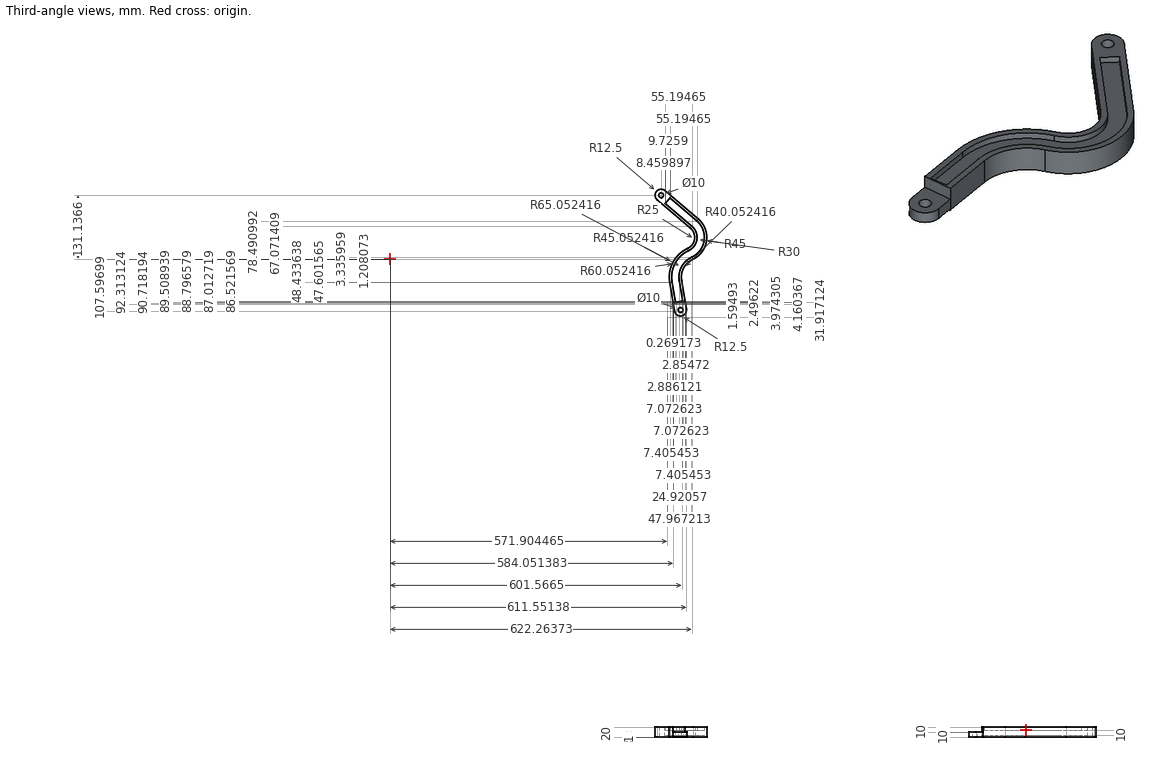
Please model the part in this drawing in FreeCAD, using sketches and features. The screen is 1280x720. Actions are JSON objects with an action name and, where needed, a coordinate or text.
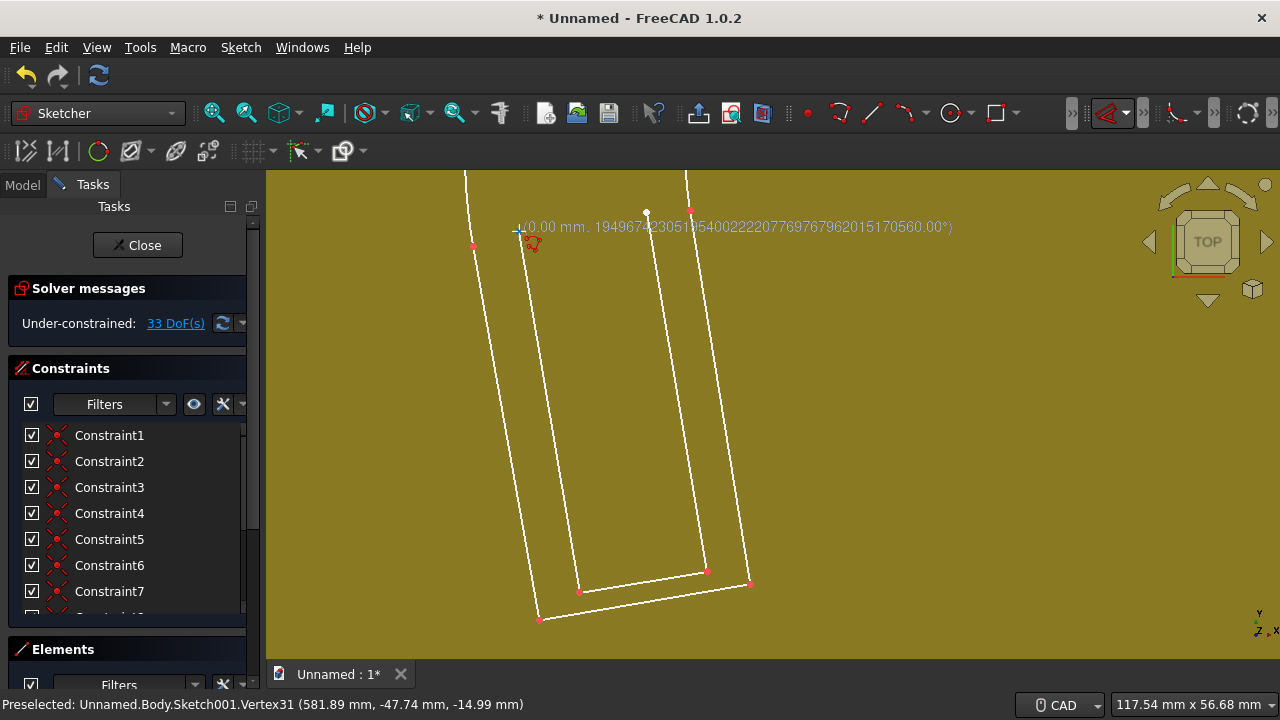
{"action": "scroll", "coordinate": [708, 573], "scroll_direction": "down", "scroll_amount": 9}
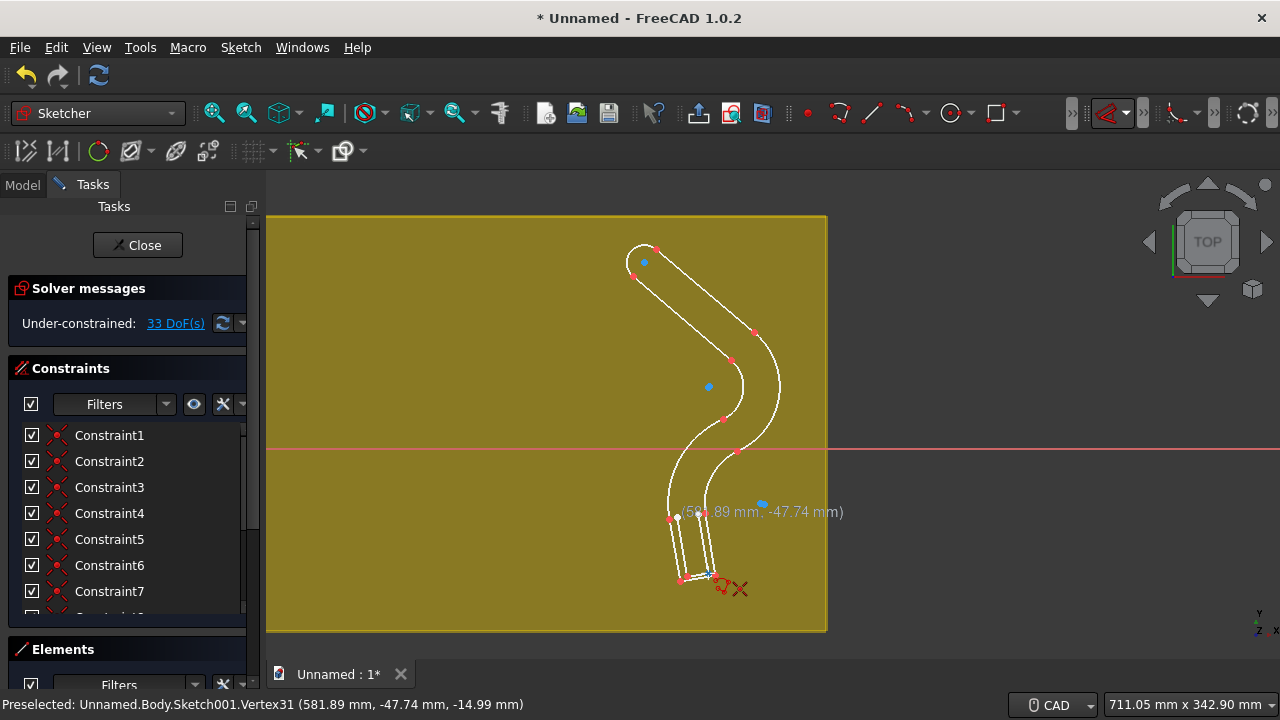
{"action": "scroll", "coordinate": [736, 354], "scroll_direction": "up", "scroll_amount": 5}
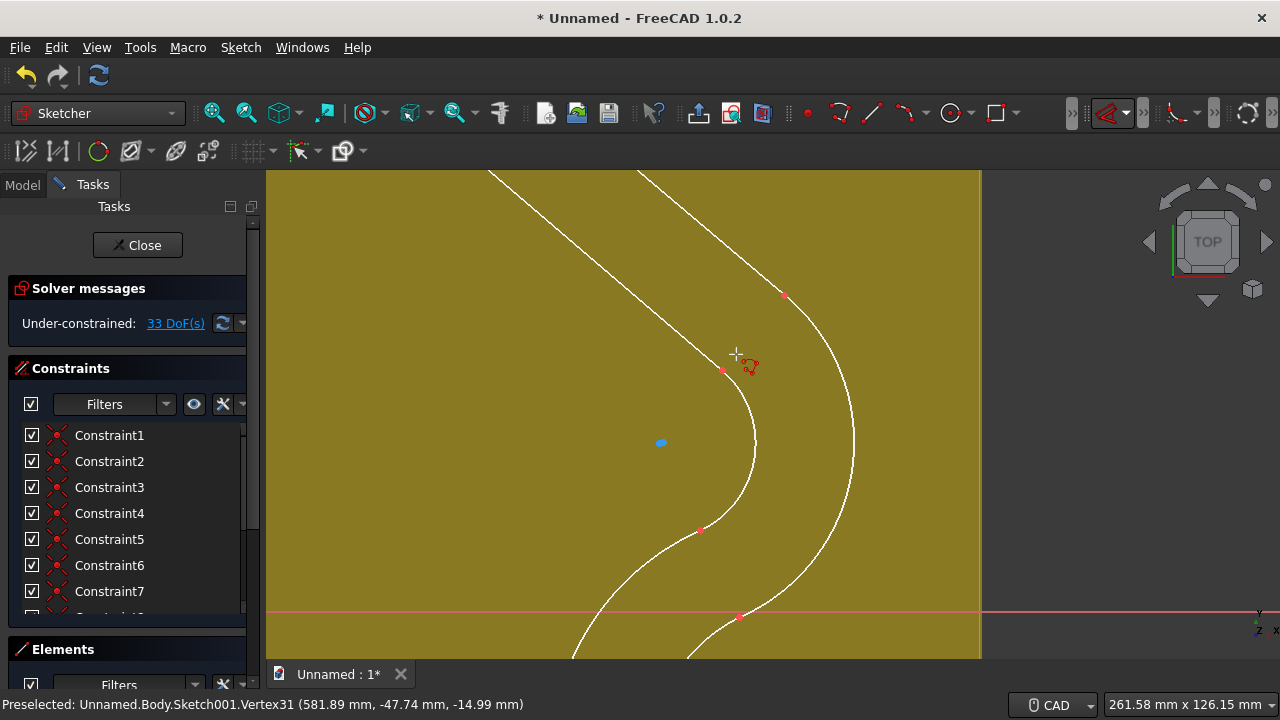
{"action": "left_click", "coordinate": [734, 352]}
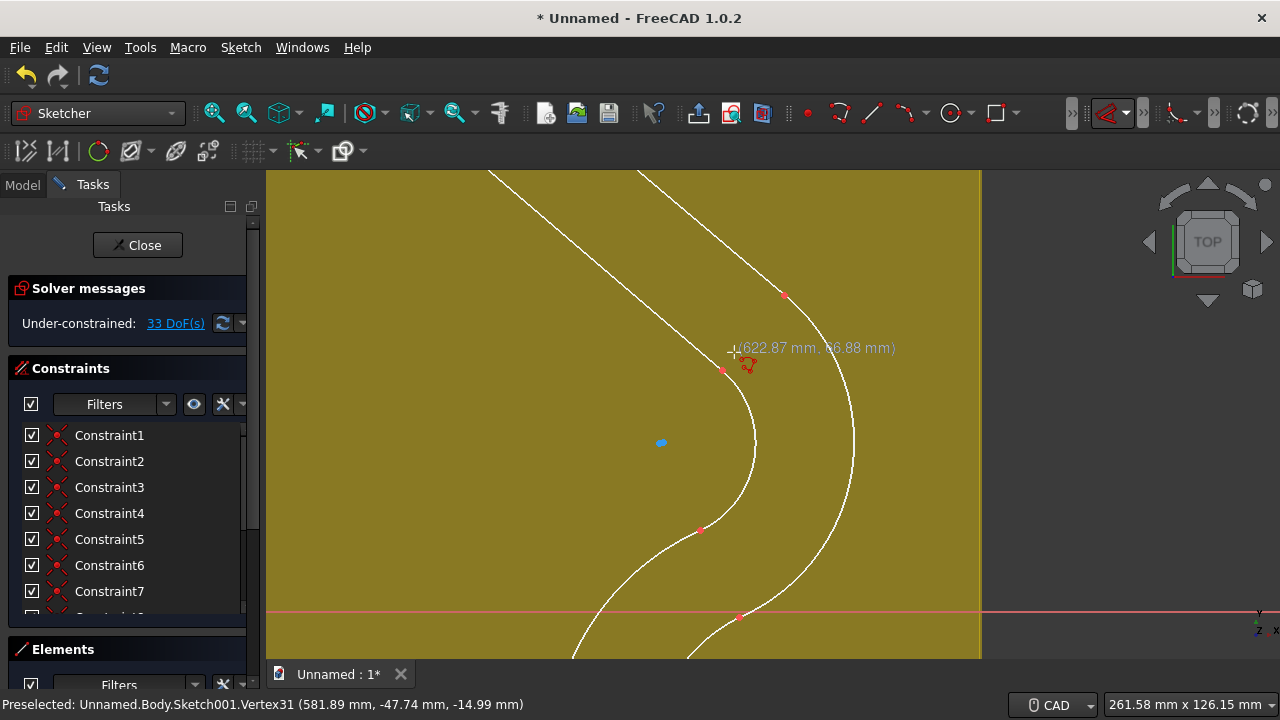
{"action": "scroll", "coordinate": [736, 354], "scroll_direction": "down", "scroll_amount": 5}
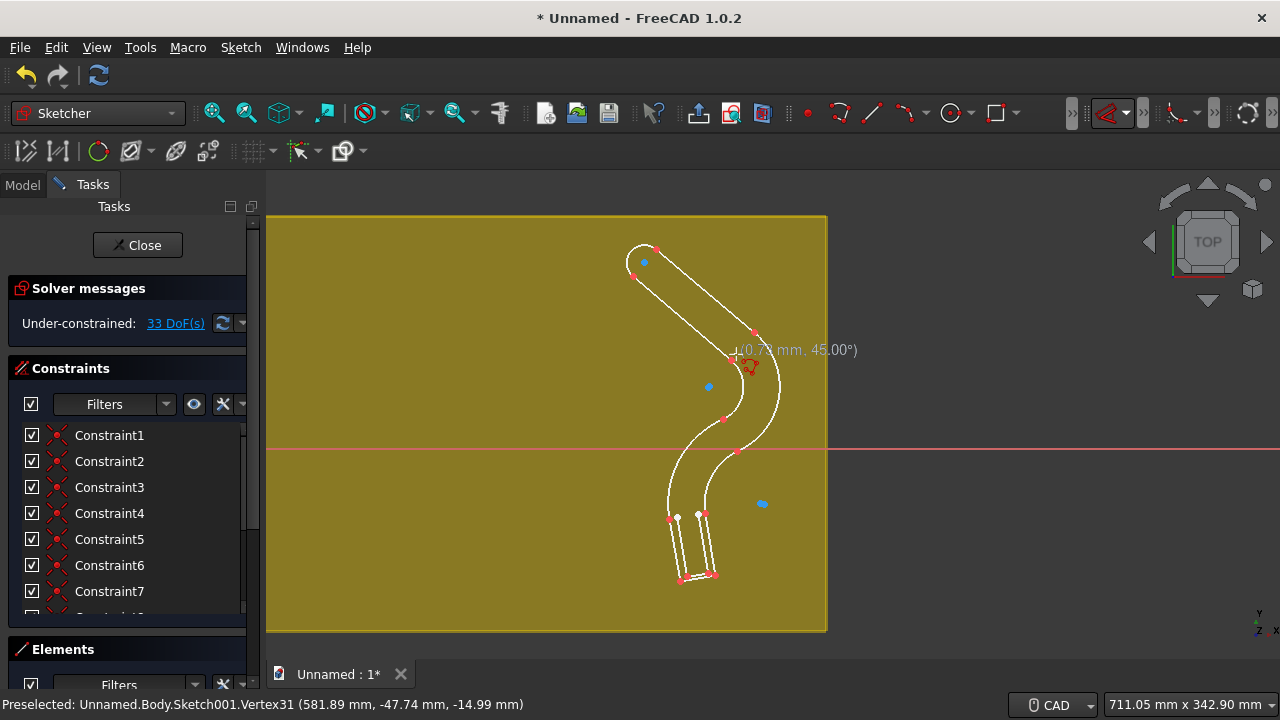
{"action": "scroll", "coordinate": [657, 287], "scroll_direction": "up", "scroll_amount": 5}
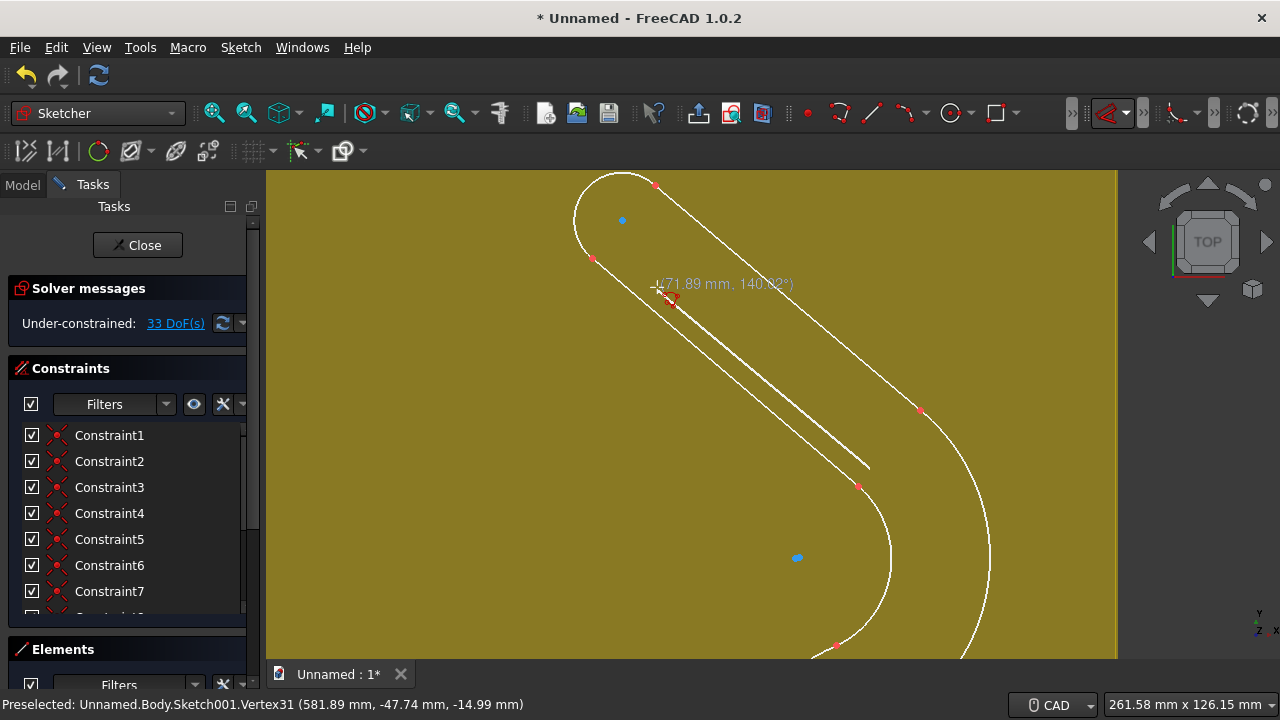
{"action": "left_click", "coordinate": [656, 285]}
{"action": "left_click", "coordinate": [694, 241]}
{"action": "left_click", "coordinate": [908, 423]}
{"action": "right_click", "coordinate": [908, 423]}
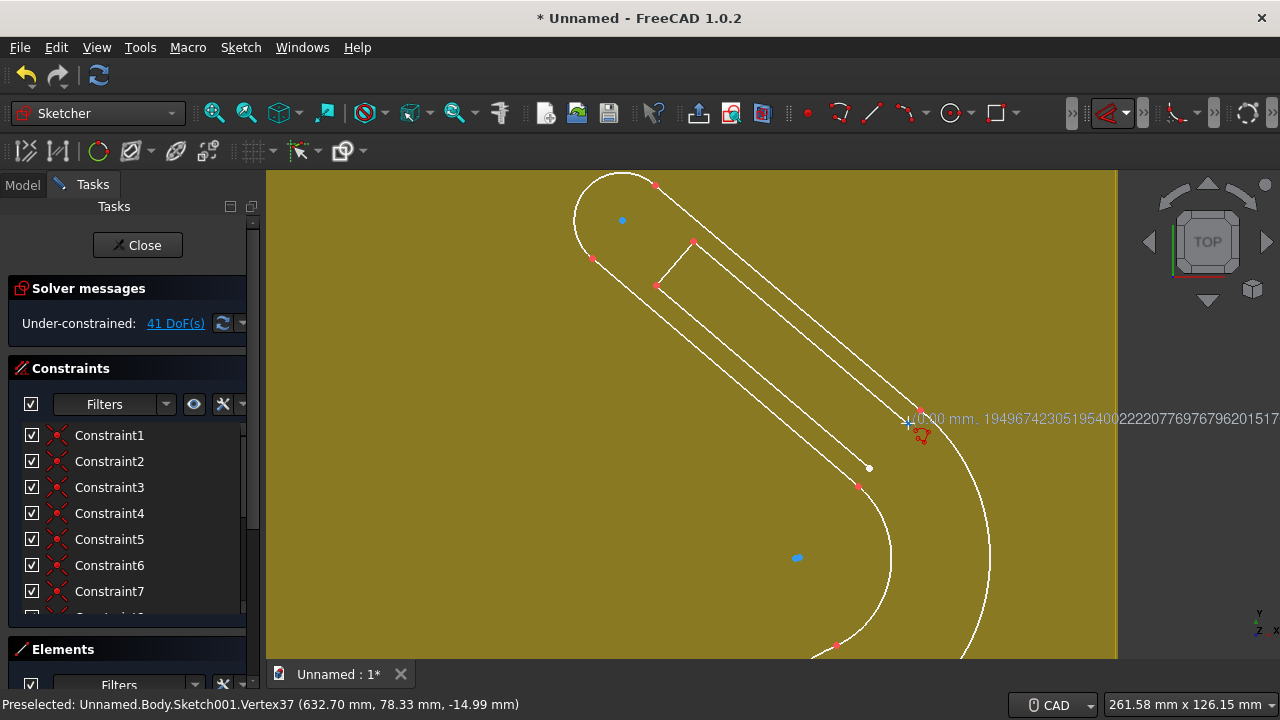
{"action": "key", "text": "g 3 a"}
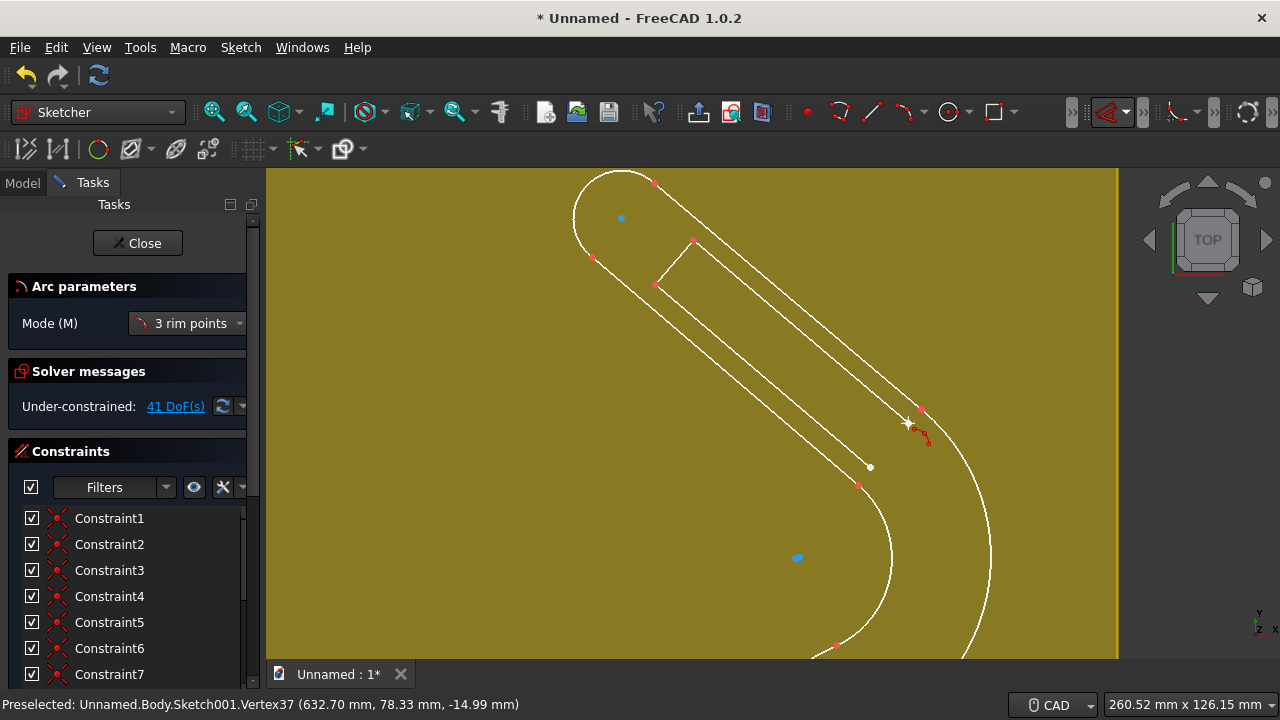
{"action": "scroll", "coordinate": [657, 285], "scroll_direction": "down", "scroll_amount": 5}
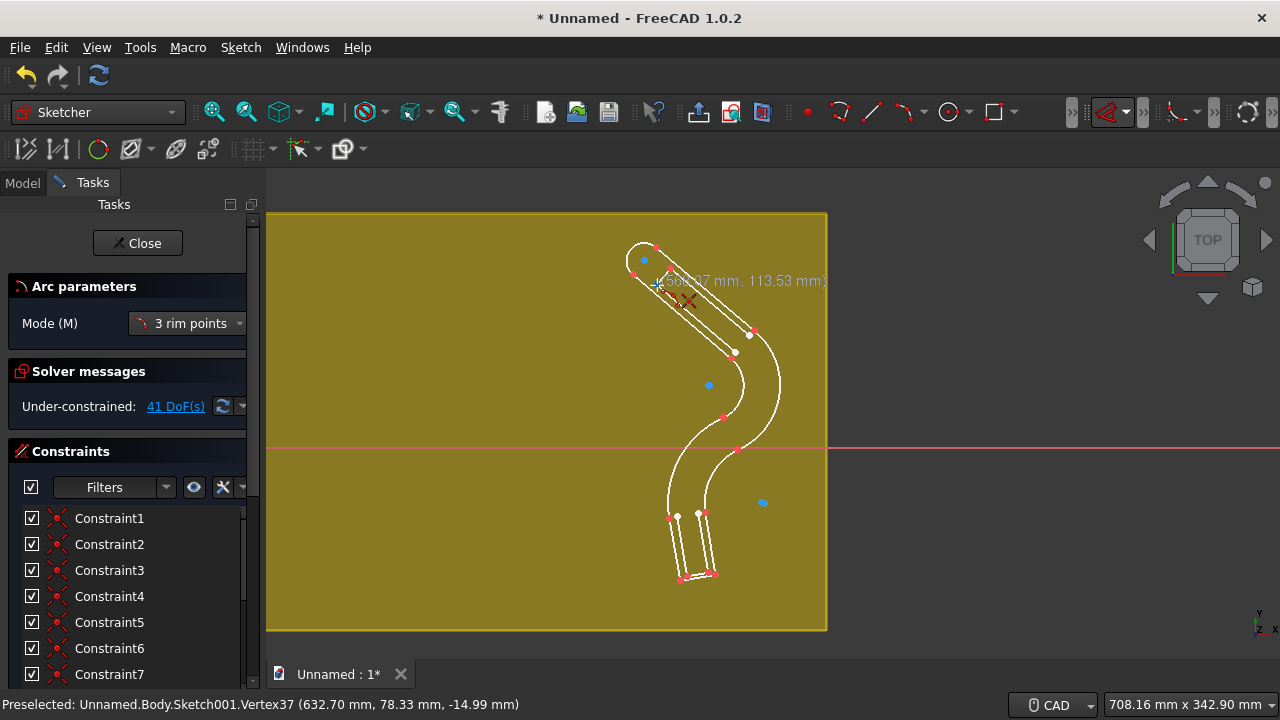
{"action": "scroll", "coordinate": [677, 516], "scroll_direction": "up", "scroll_amount": 4}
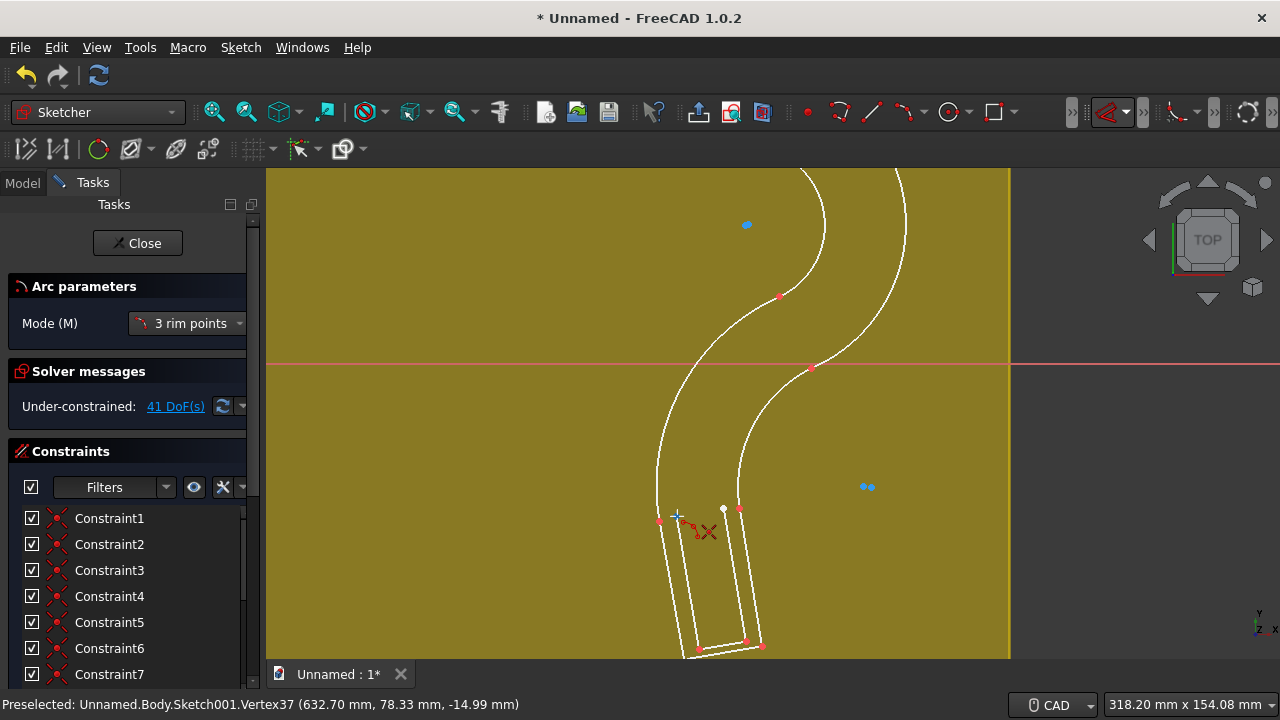
{"action": "left_click", "coordinate": [677, 516]}
{"action": "left_click", "coordinate": [785, 310]}
{"action": "left_click", "coordinate": [679, 441]}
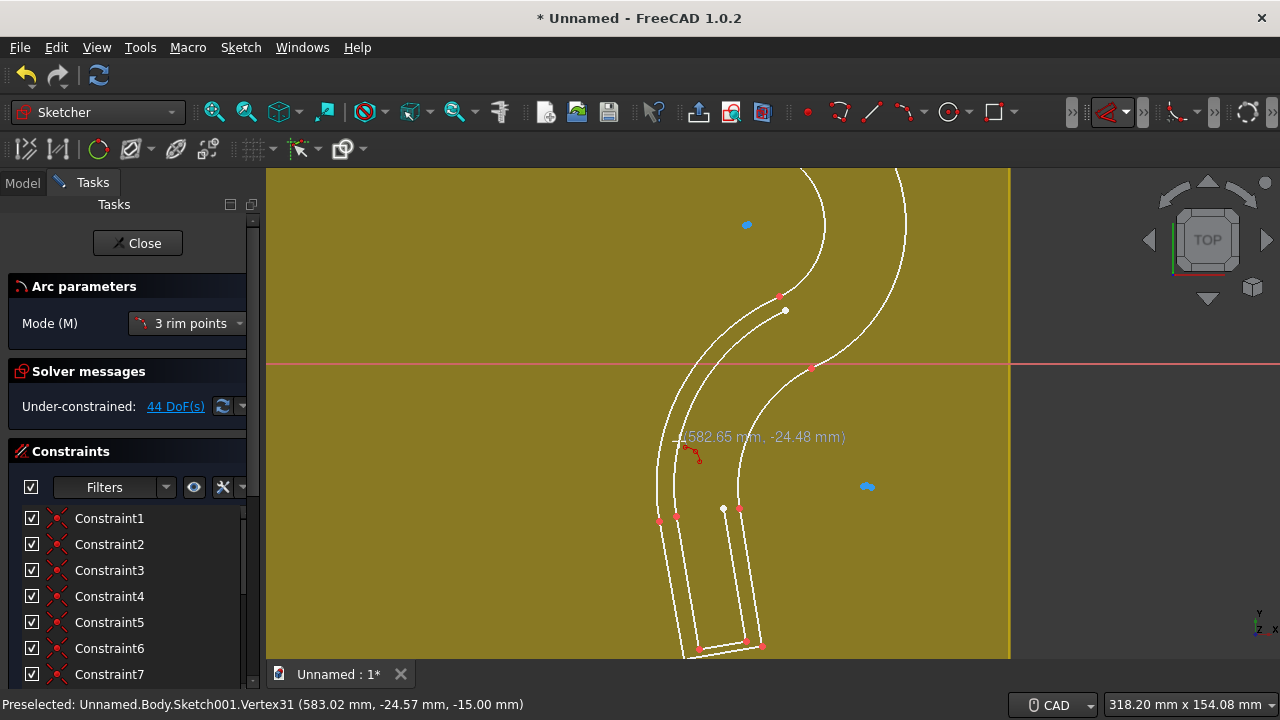
{"action": "left_click", "coordinate": [785, 311]}